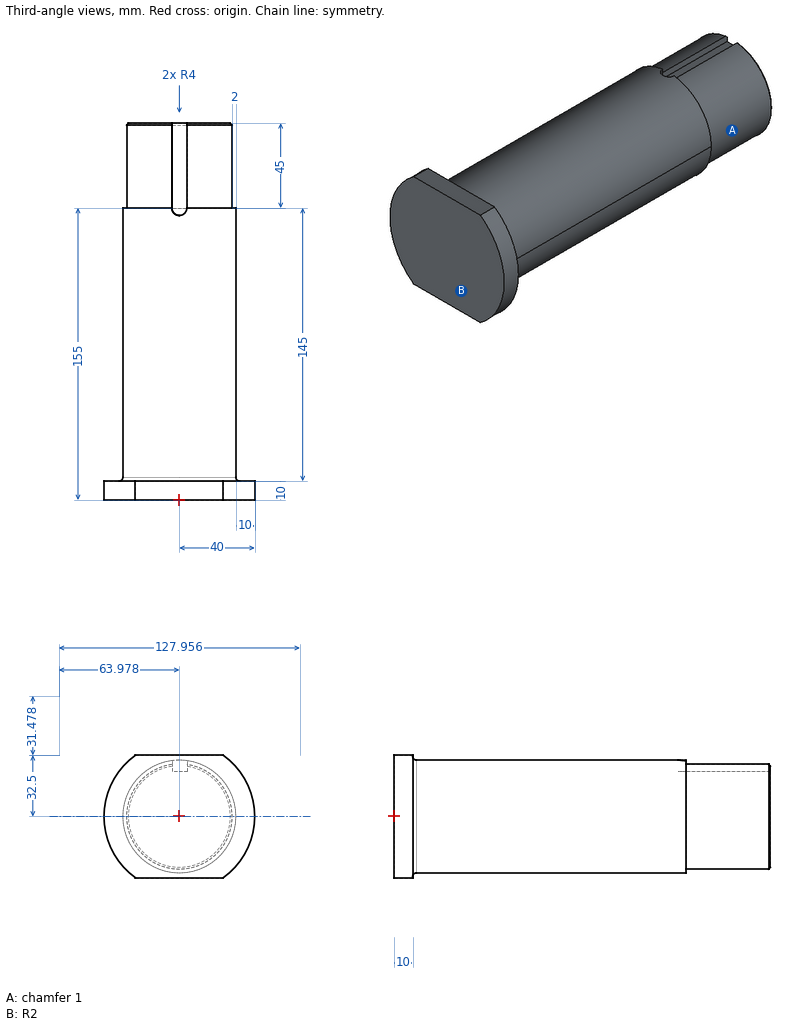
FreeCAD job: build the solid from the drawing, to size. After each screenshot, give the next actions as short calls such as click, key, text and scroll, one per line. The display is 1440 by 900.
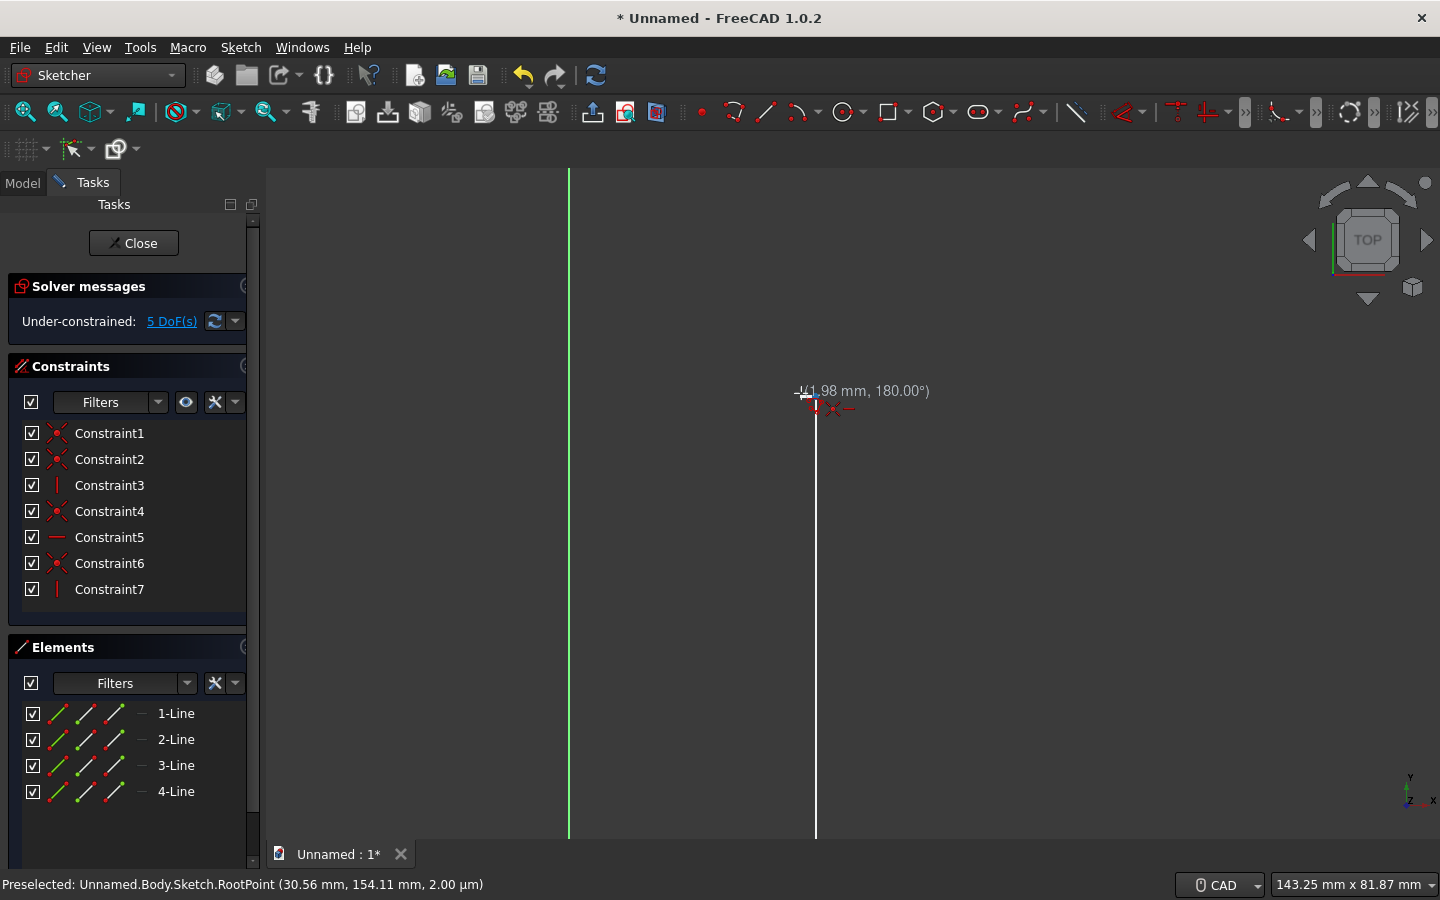
click(799, 392)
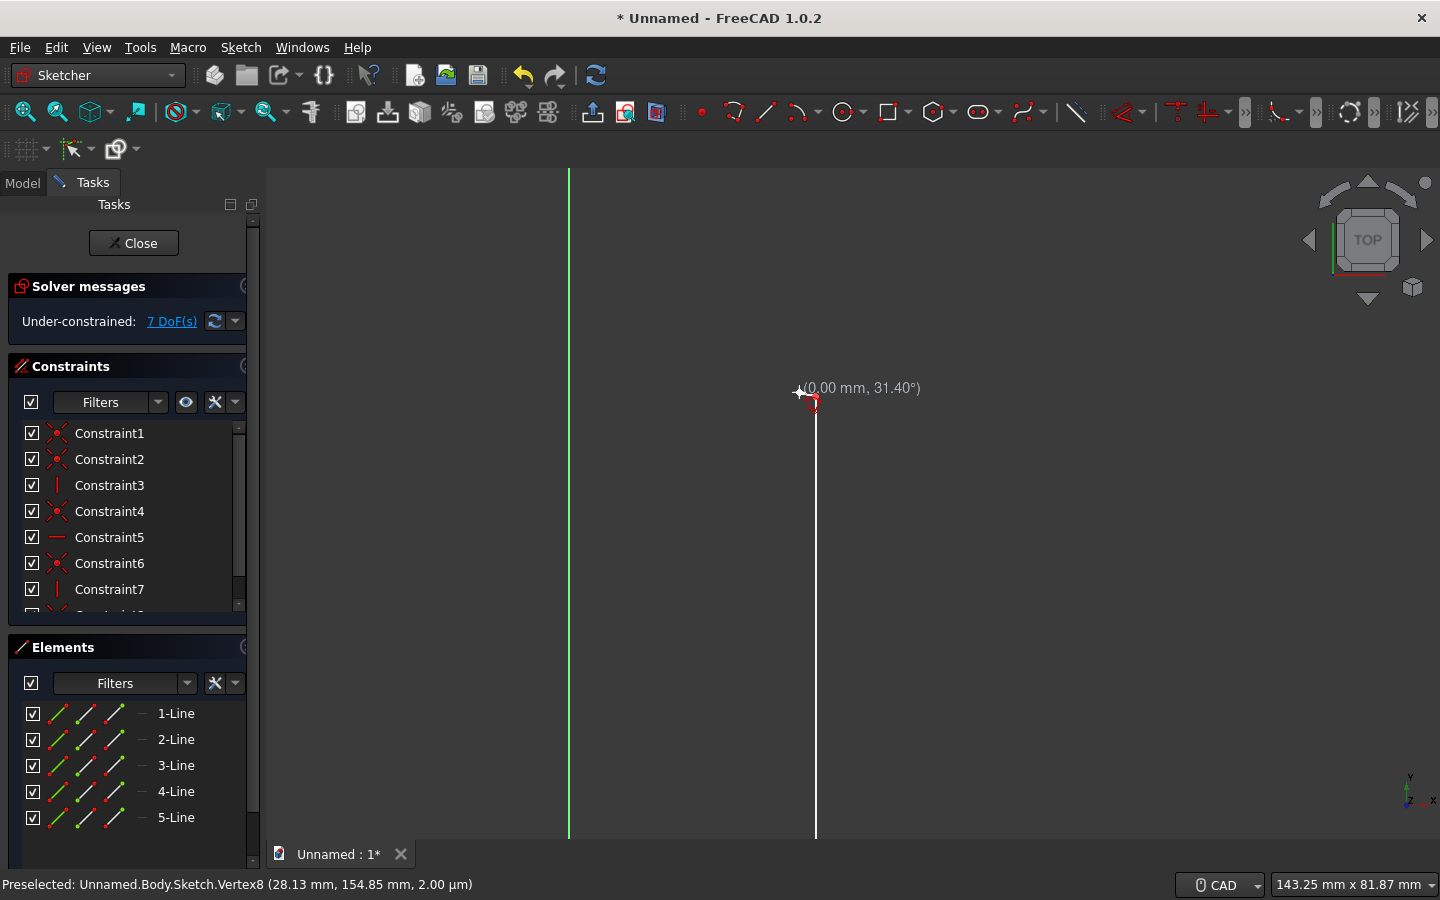
scroll(801, 392, down, 7)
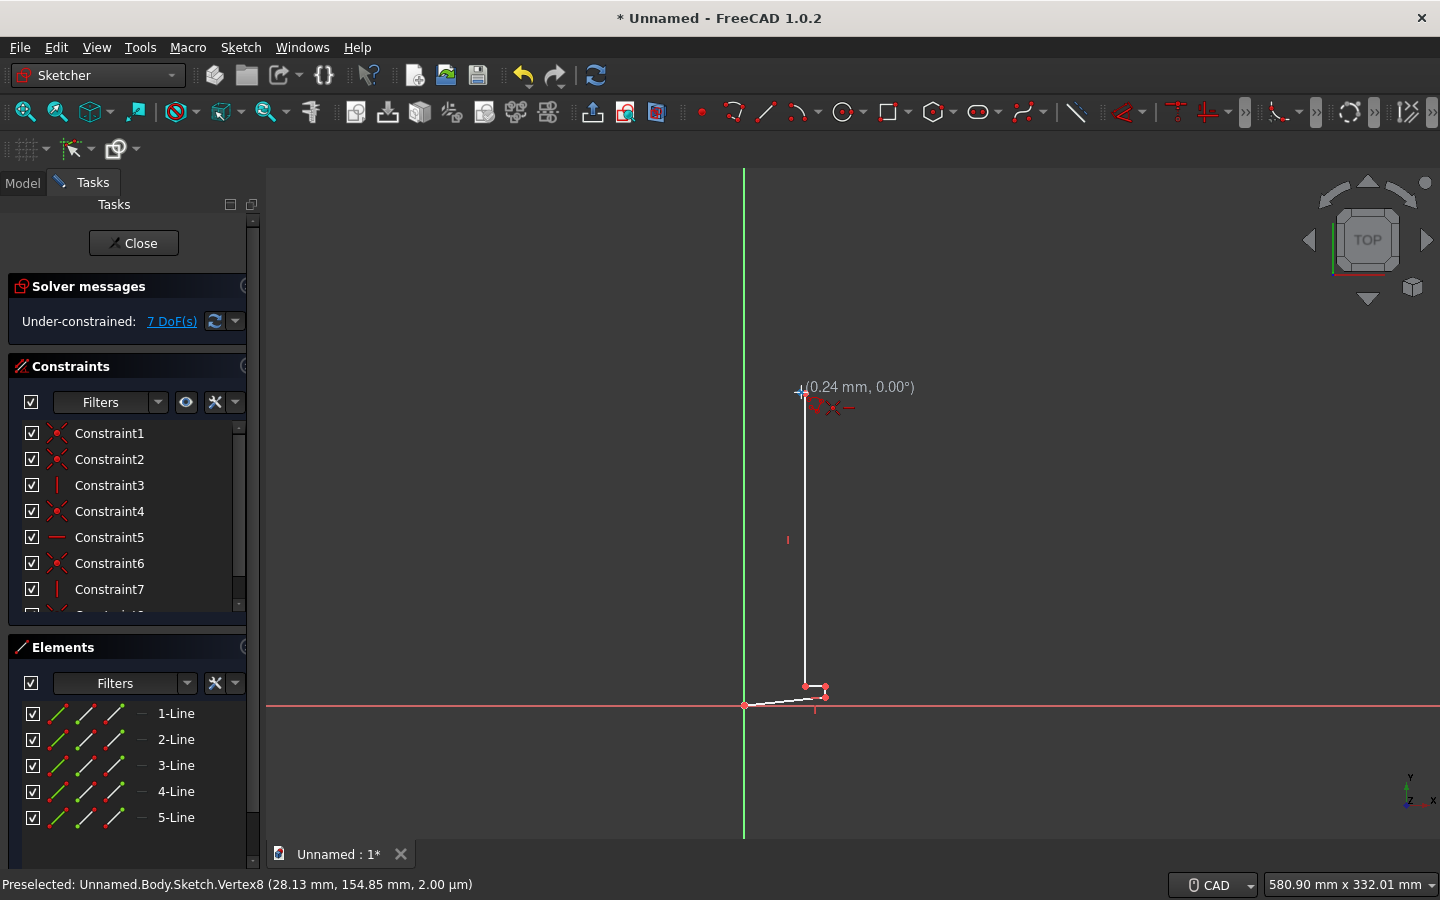
click(801, 301)
click(753, 301)
click(744, 706)
key(Escape)
key(Escape)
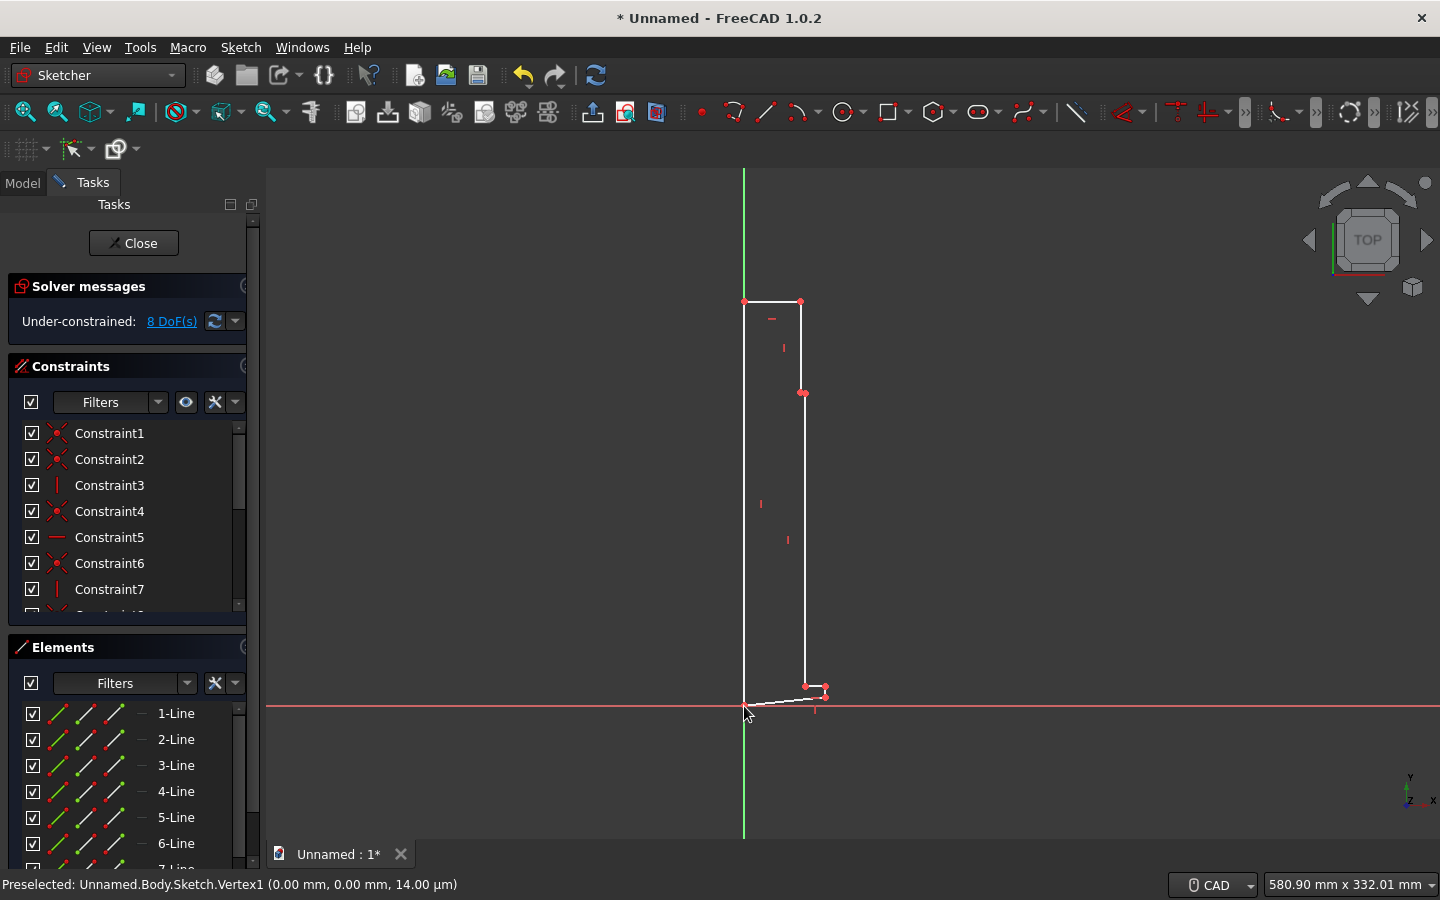
click(768, 703)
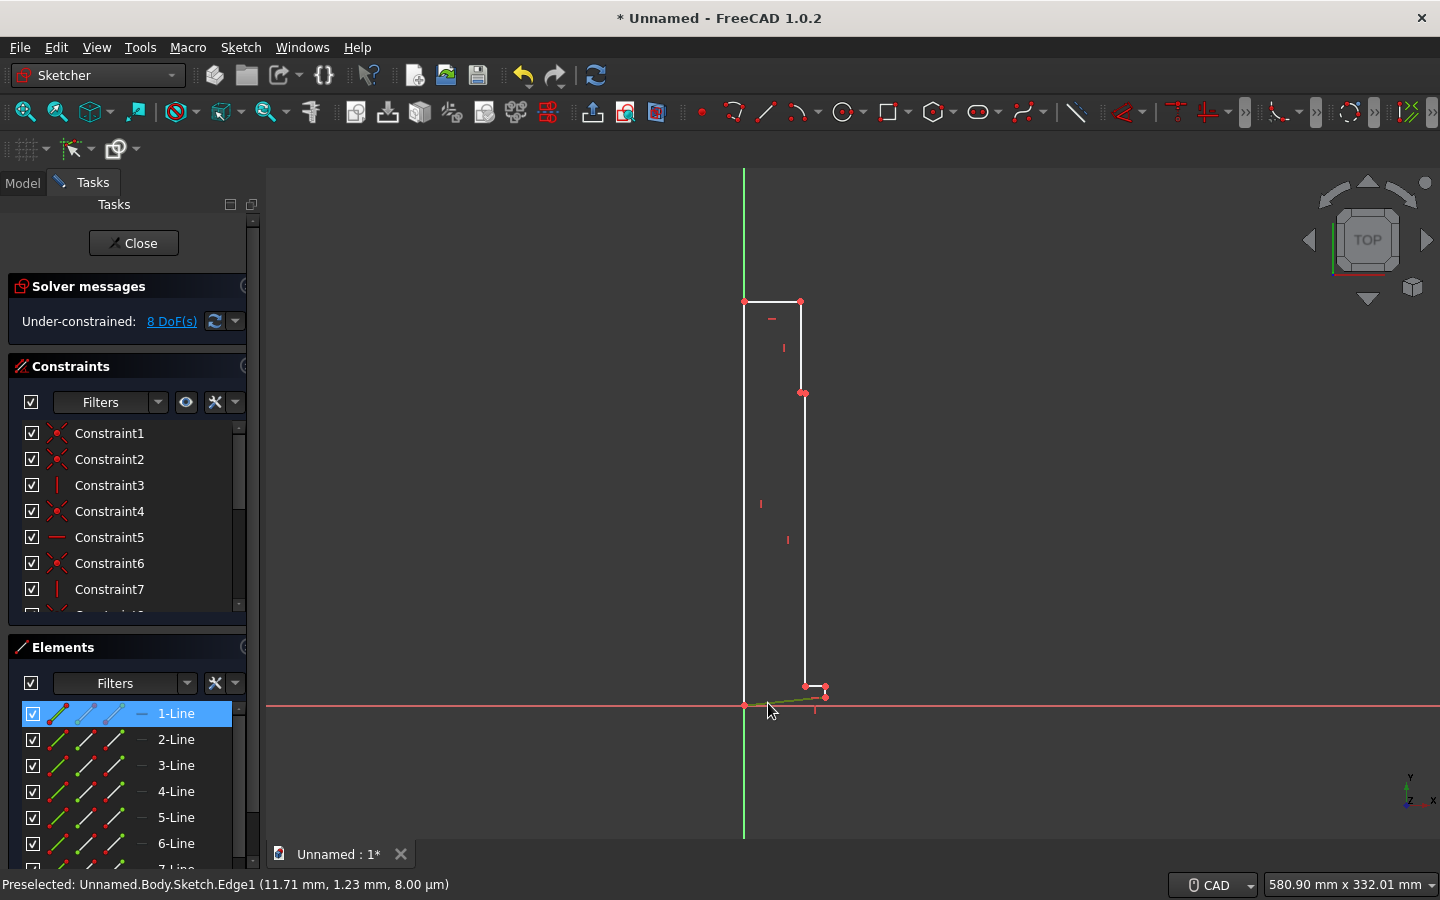
key(h)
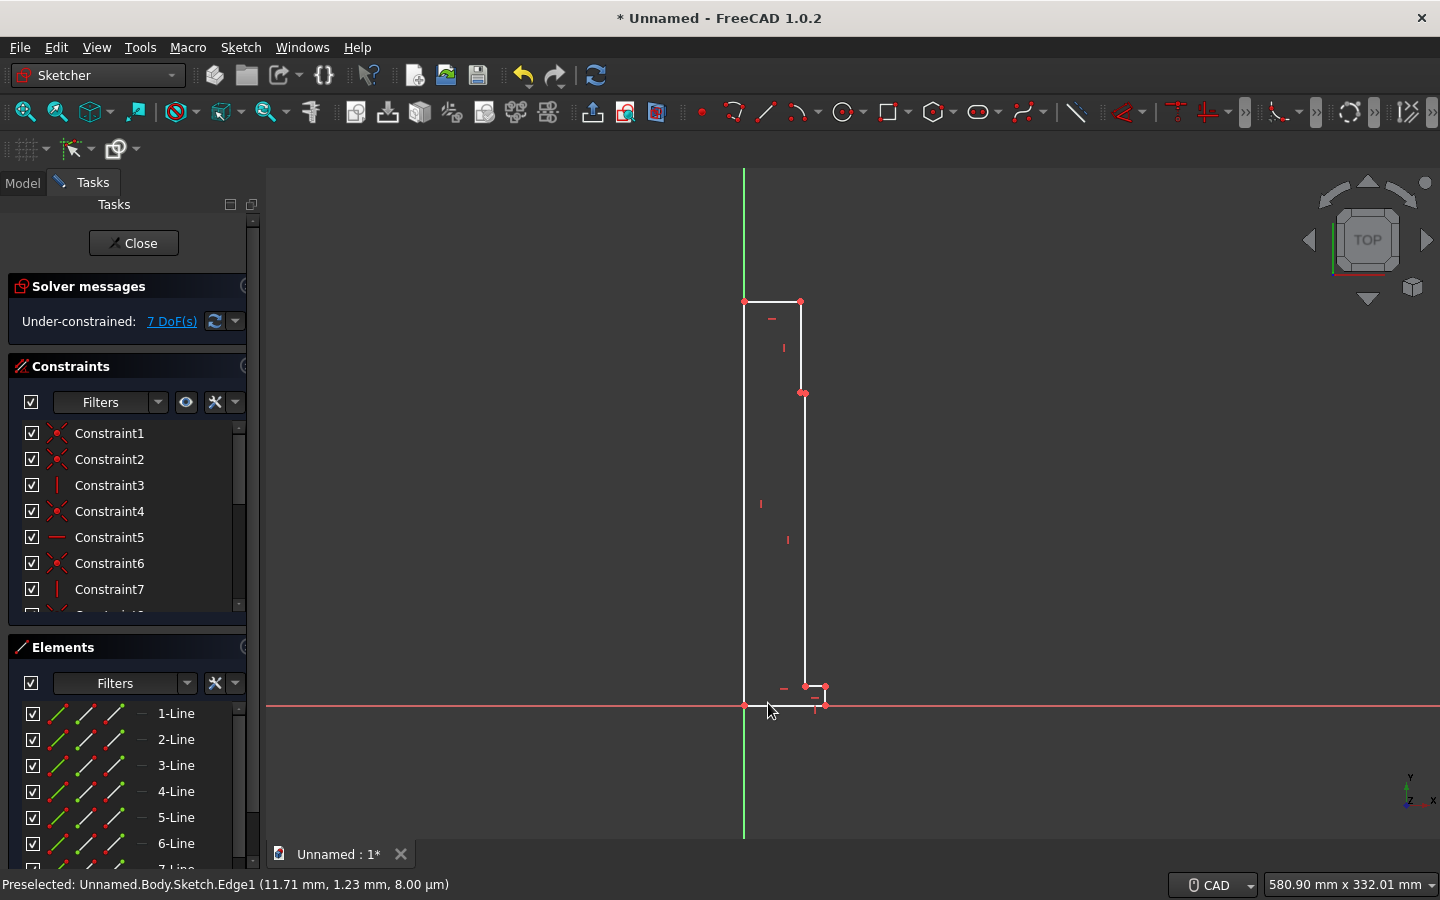
scroll(803, 393, up, 10)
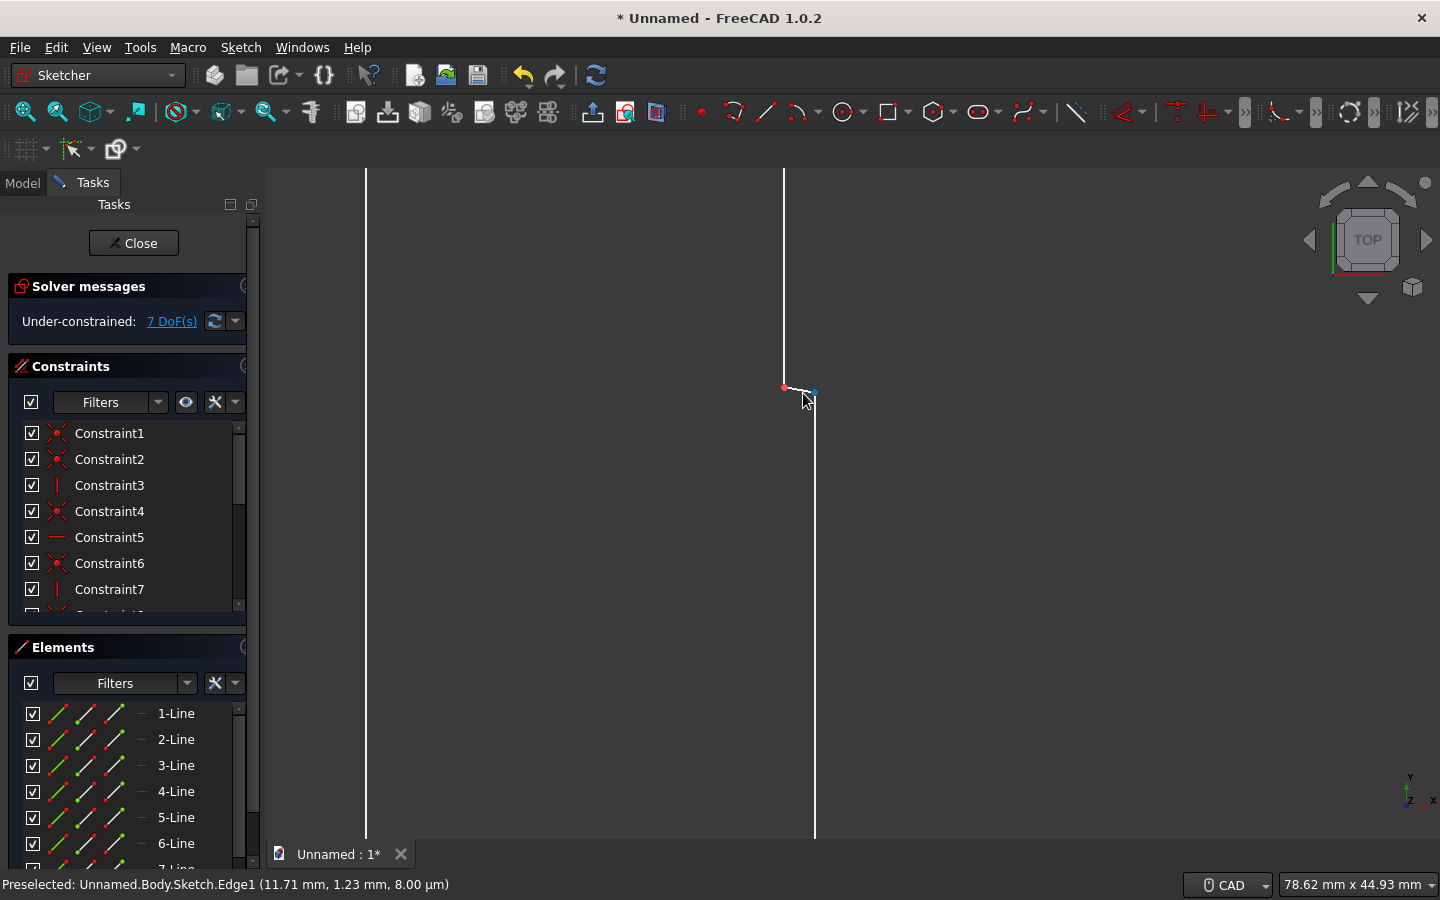
click(800, 390)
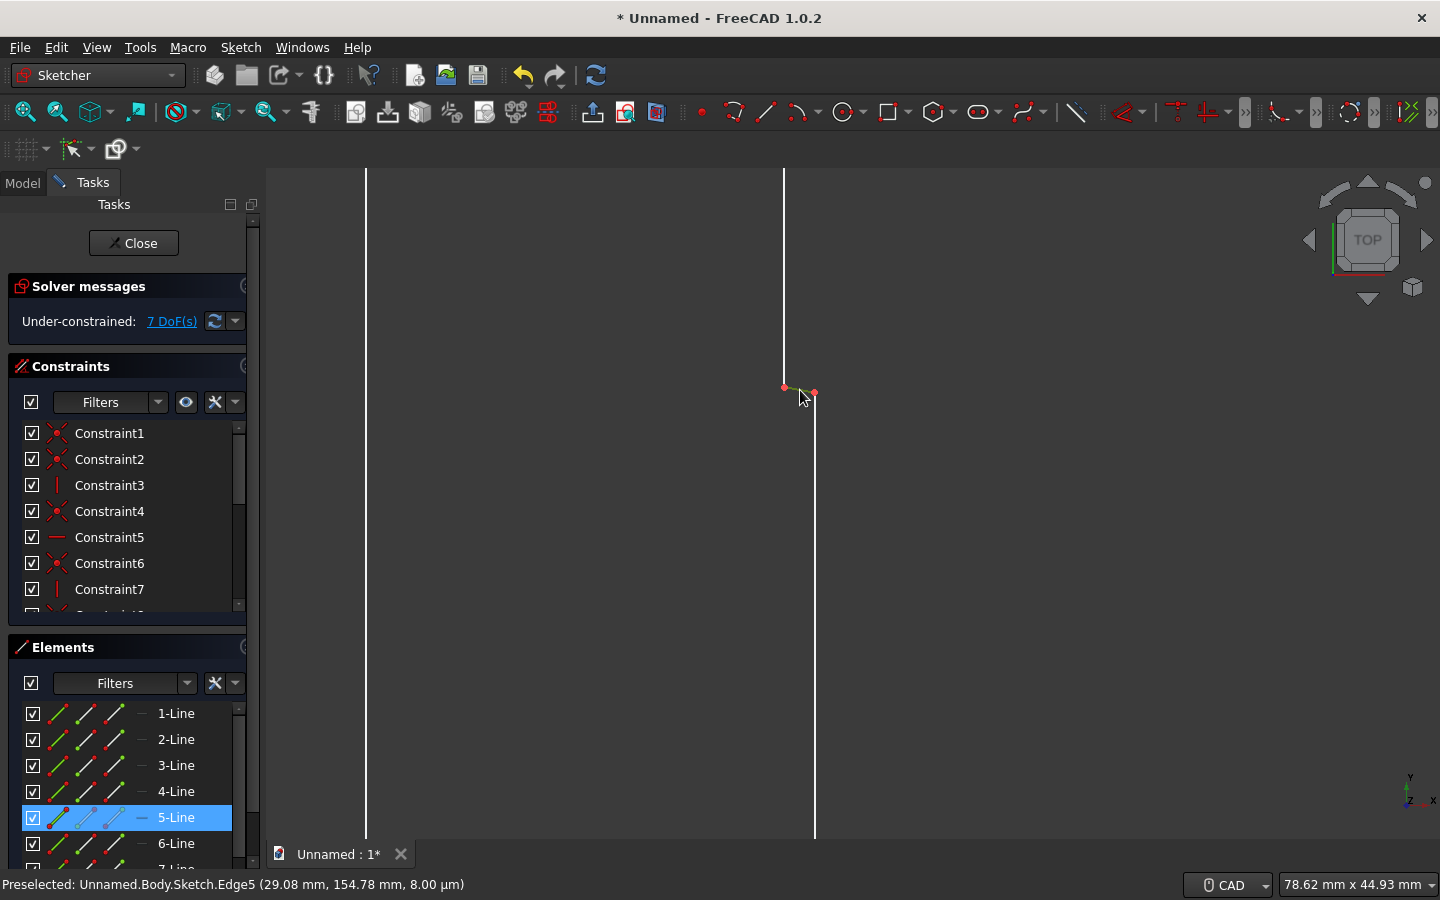
click(1230, 112)